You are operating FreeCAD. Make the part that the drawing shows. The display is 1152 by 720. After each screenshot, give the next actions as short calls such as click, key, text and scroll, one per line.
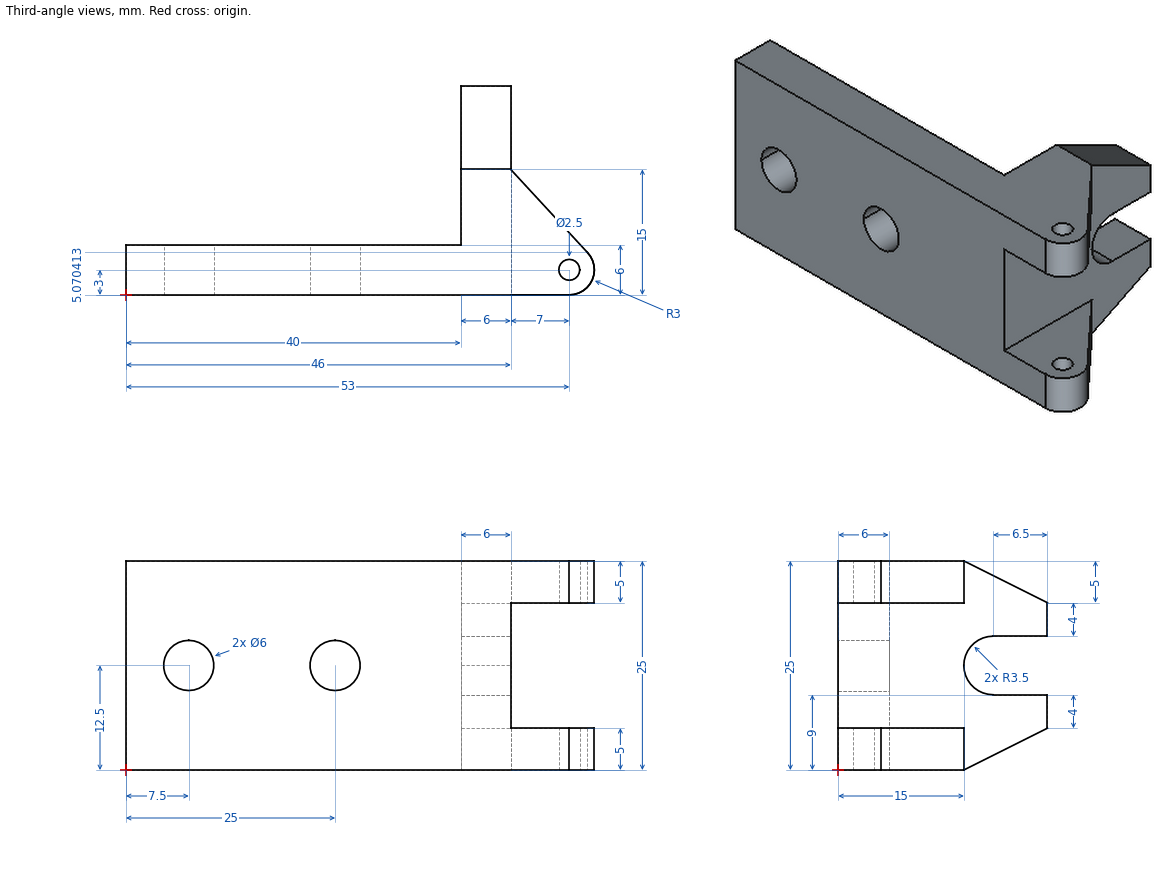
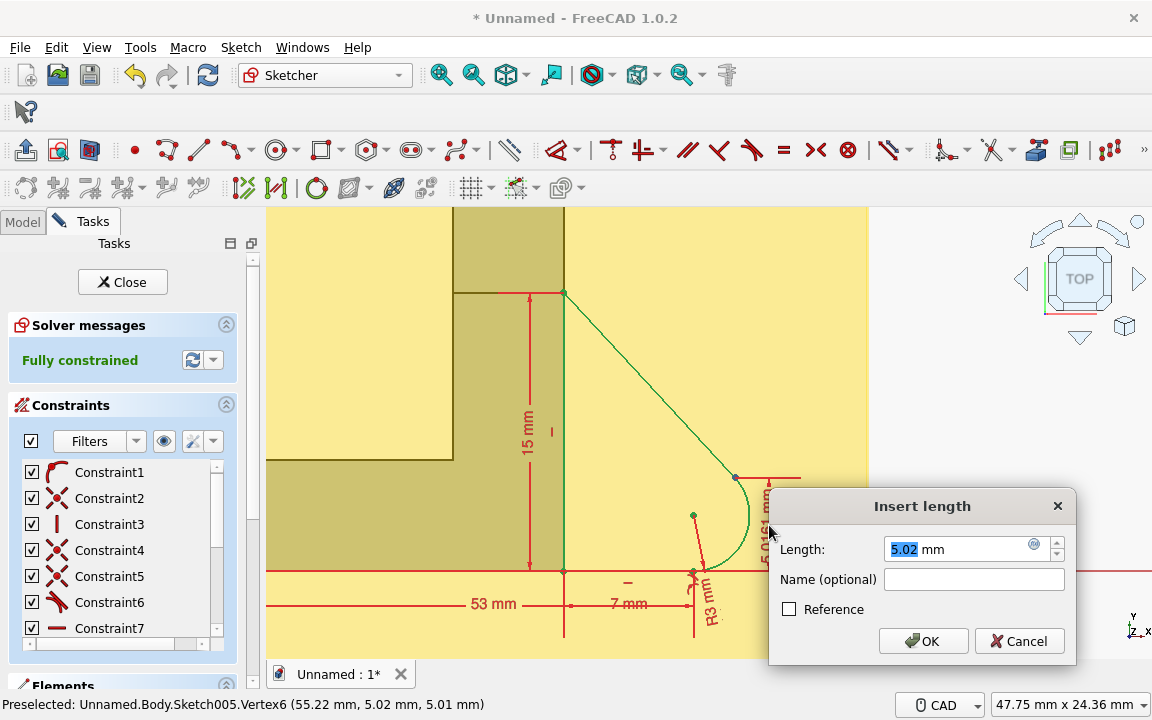
text(5.070413)
key(Return)
key(Escape)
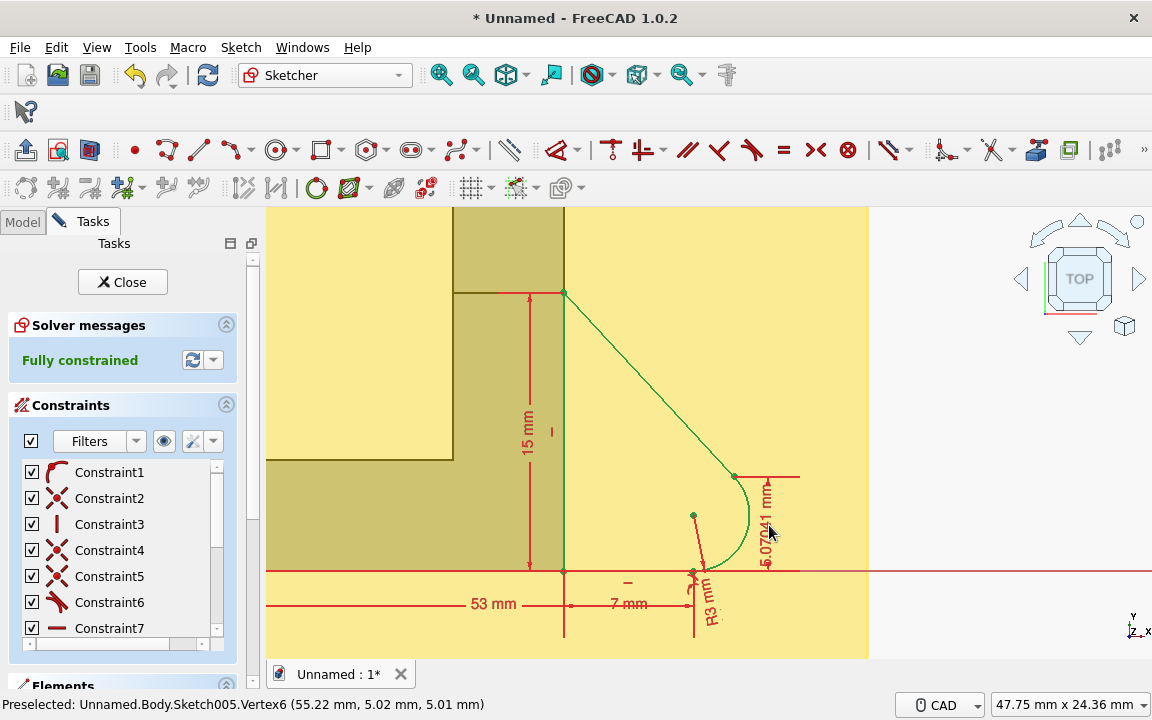
click(123, 282)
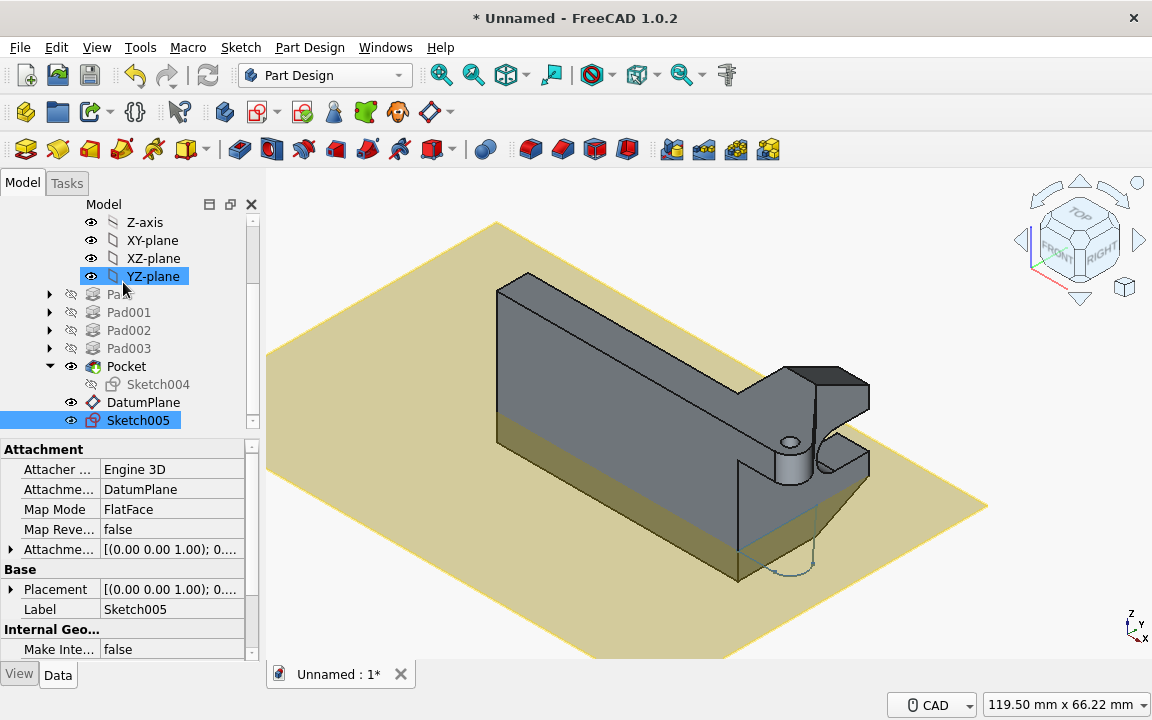
click(26, 150)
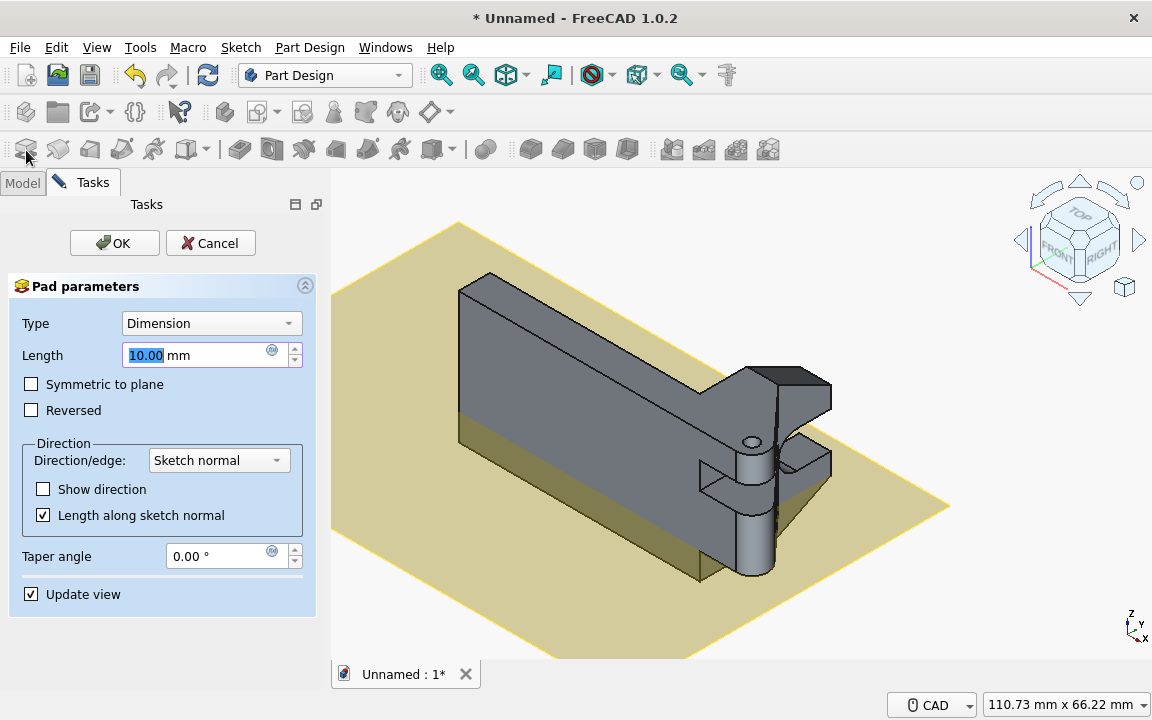
text(5)
key(Tab)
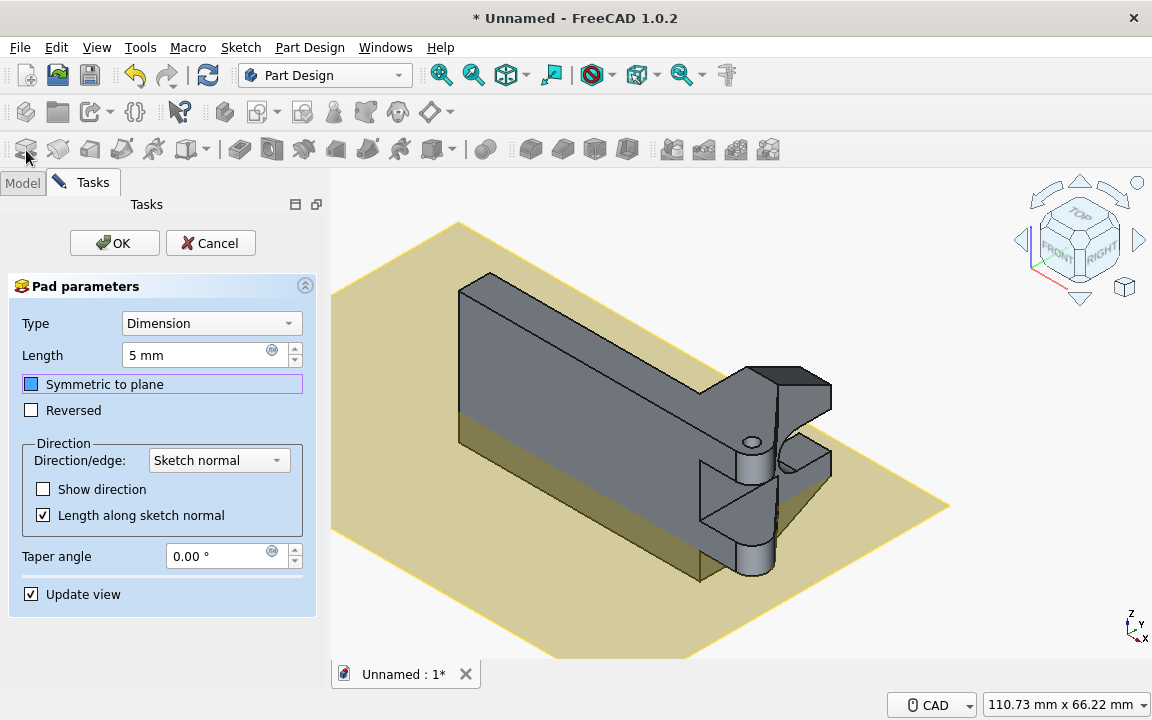
click(30, 410)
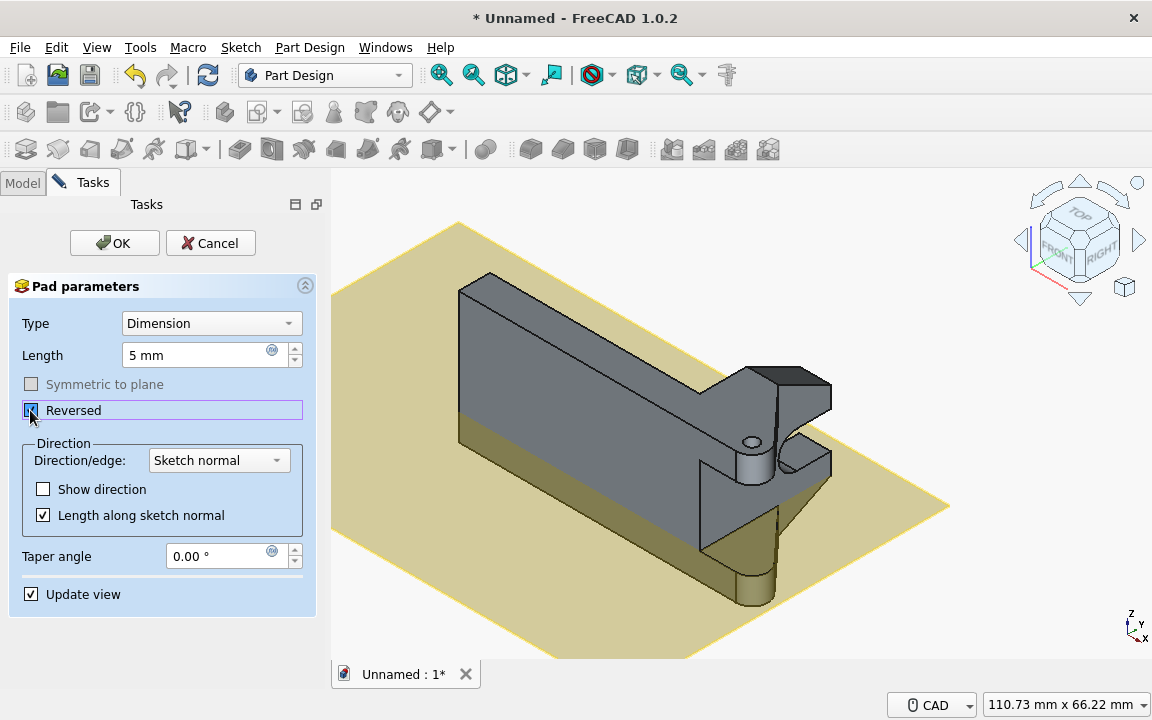
click(115, 243)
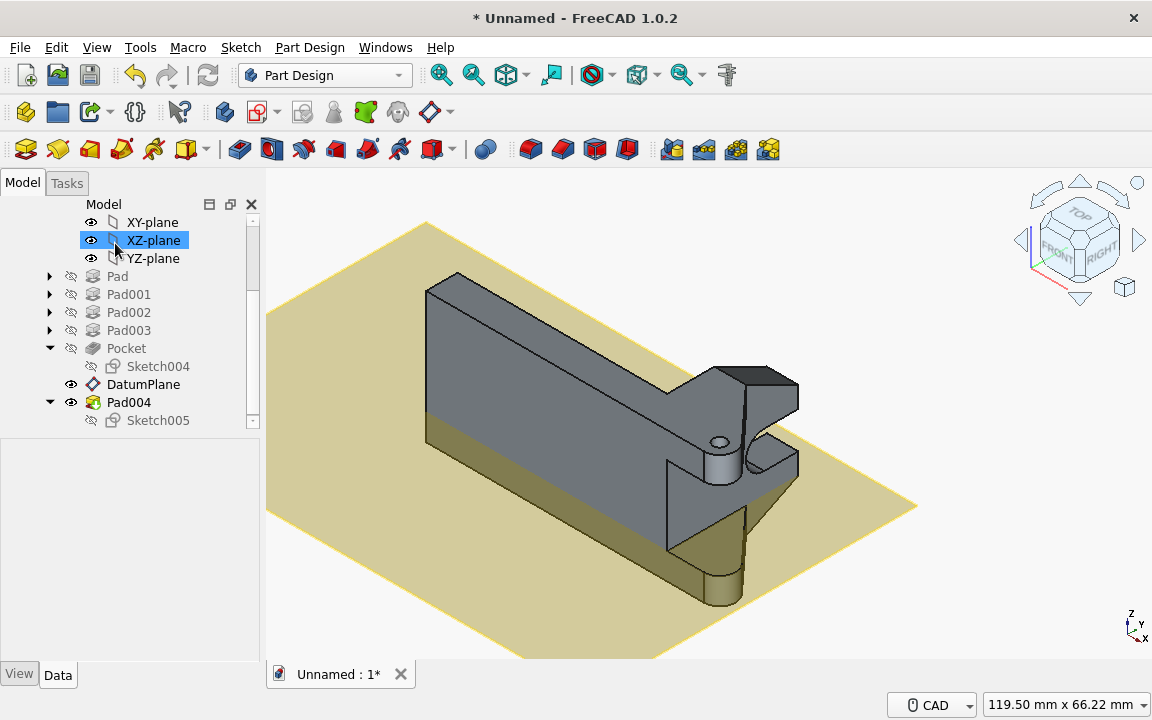
click(116, 384)
key(space)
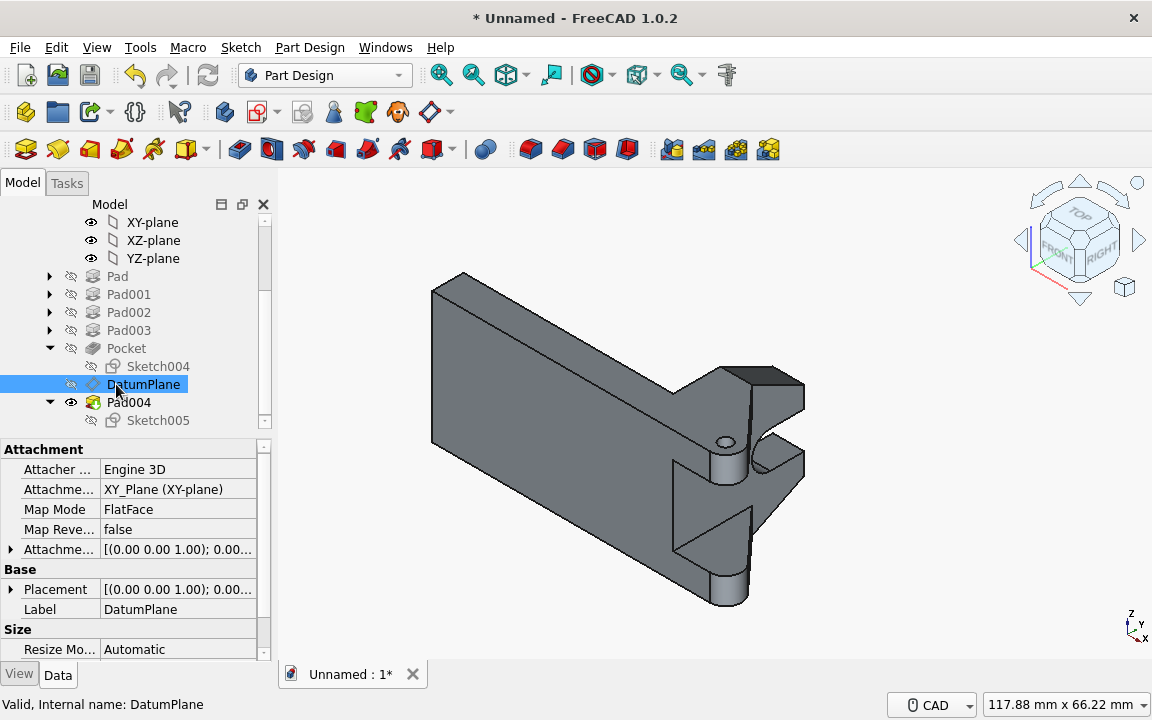
click(724, 560)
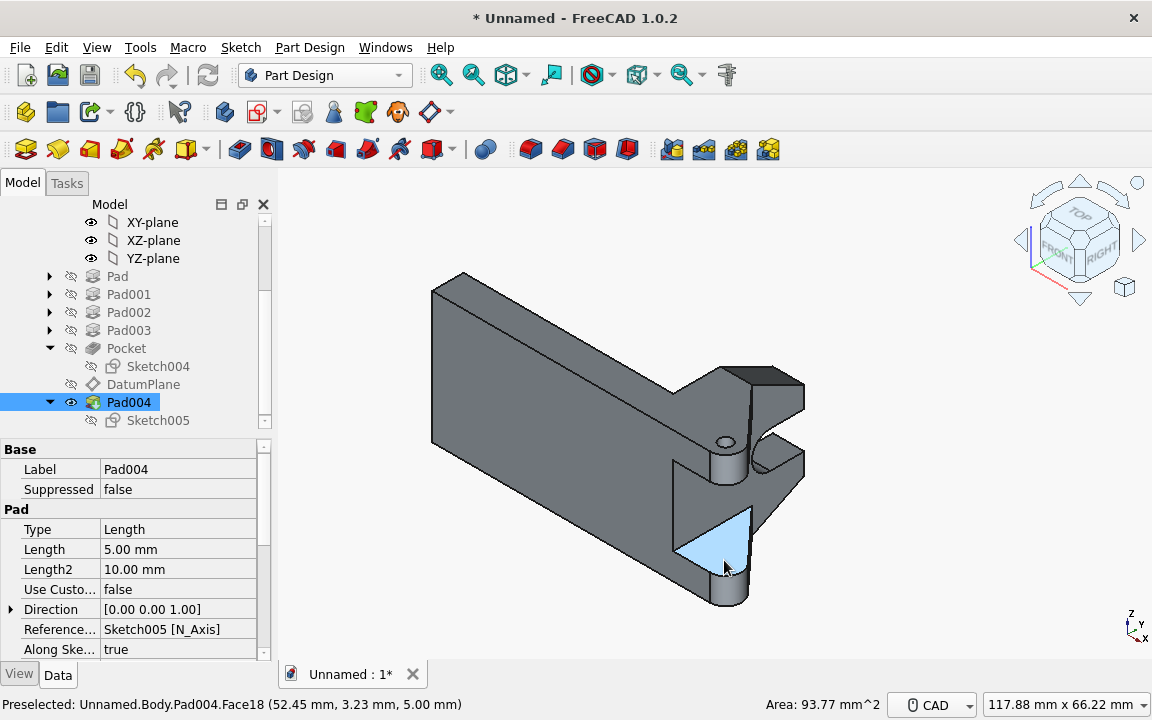
click(258, 112)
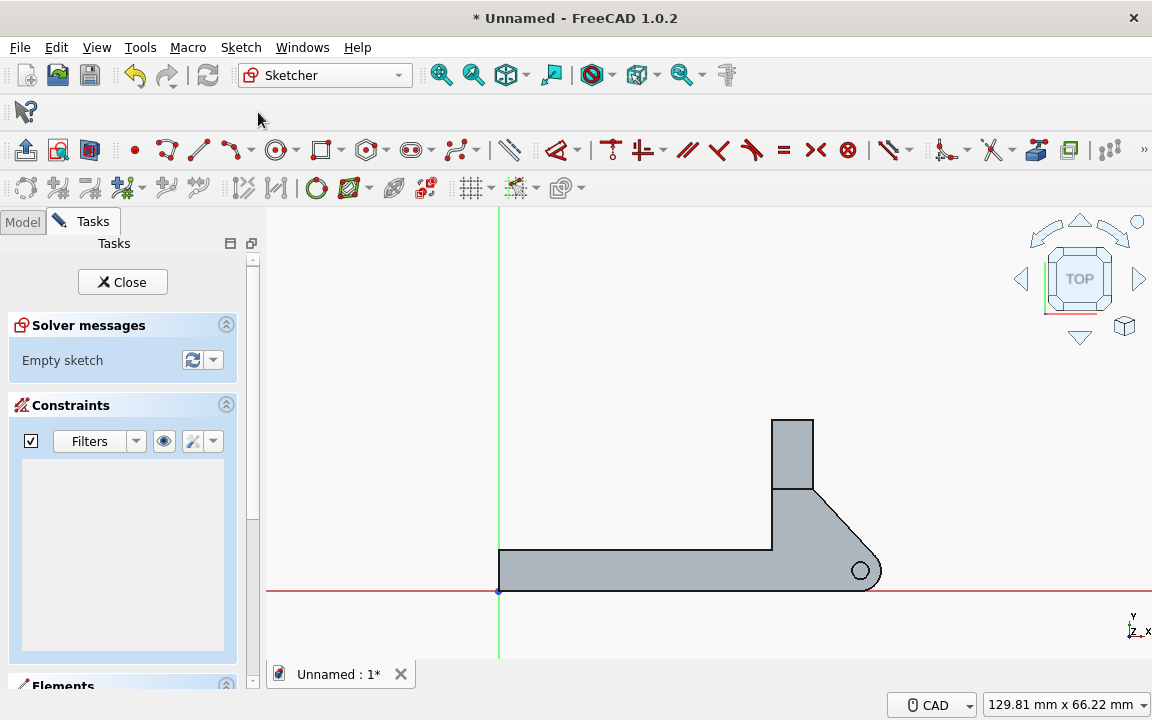
key(q)
key(s)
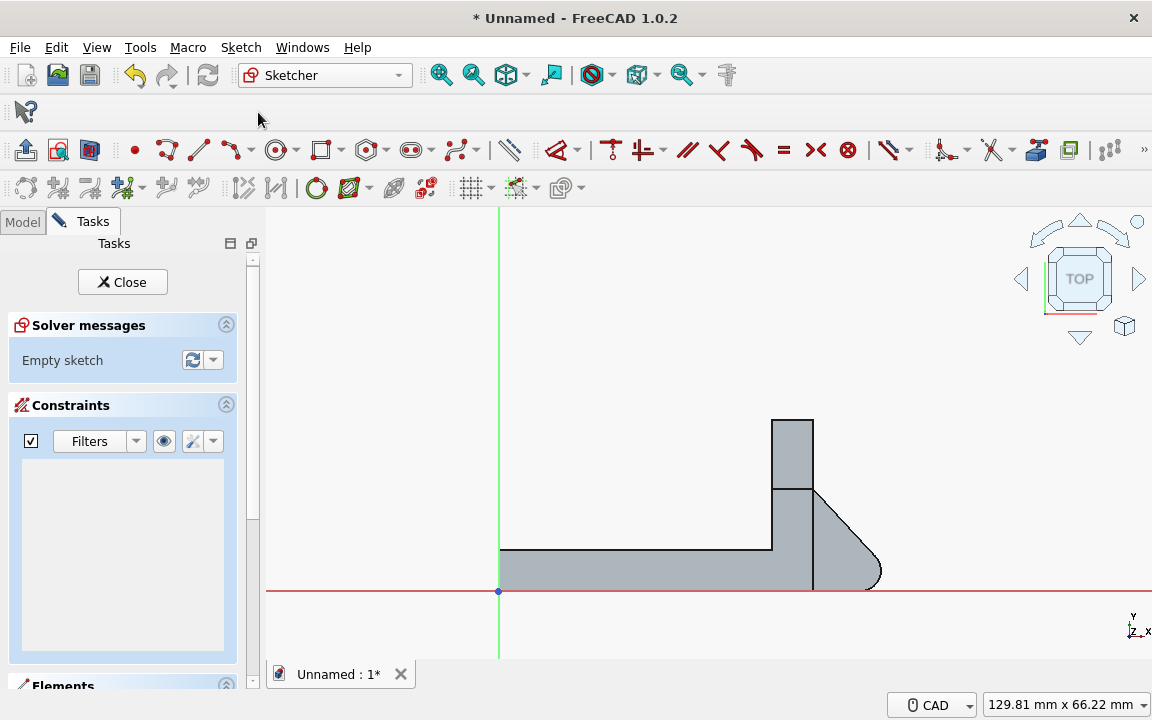
scroll(875, 580, up, 14)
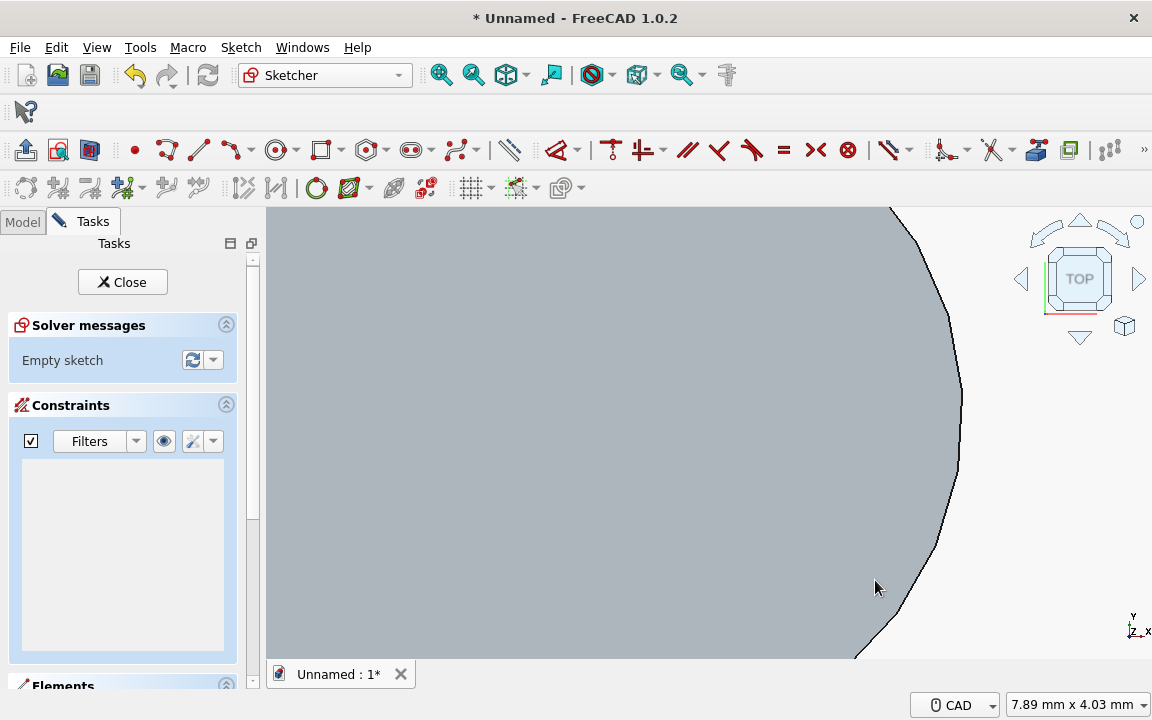
key(g)
key(c)